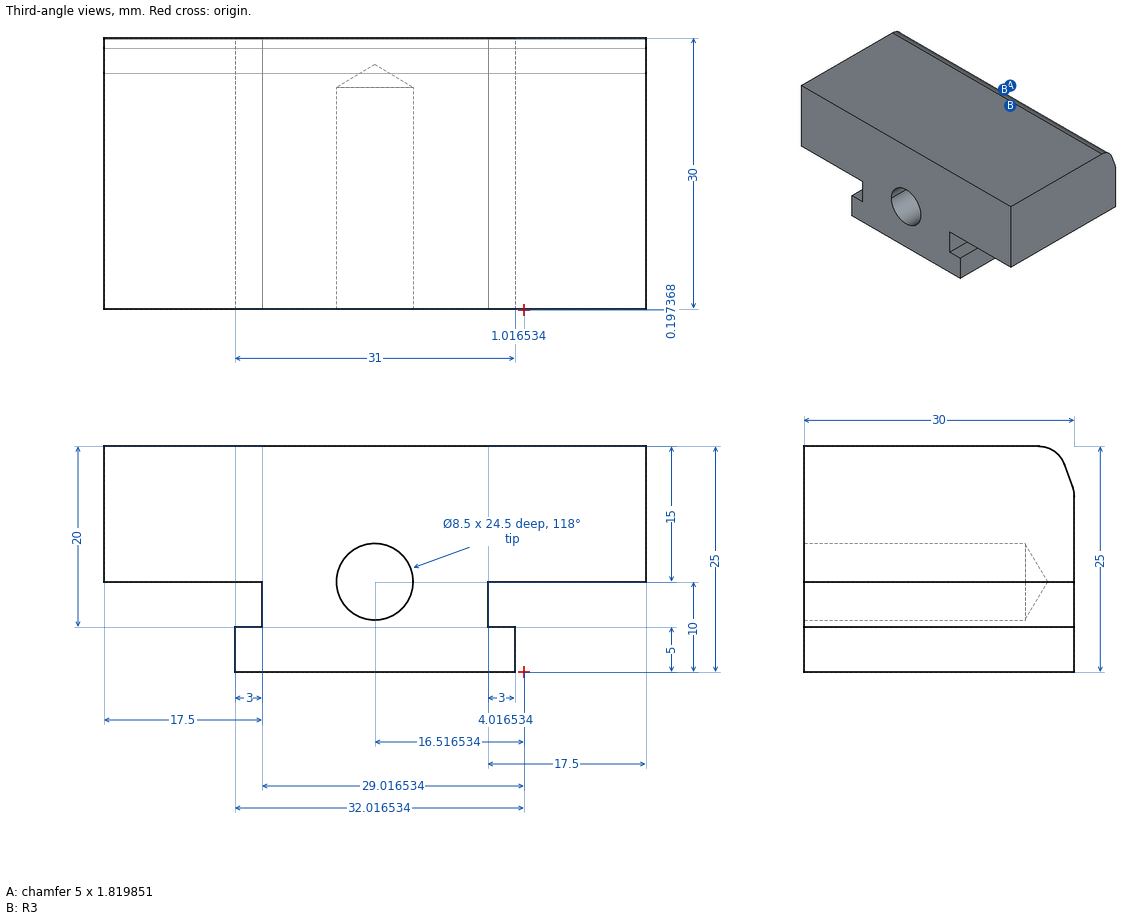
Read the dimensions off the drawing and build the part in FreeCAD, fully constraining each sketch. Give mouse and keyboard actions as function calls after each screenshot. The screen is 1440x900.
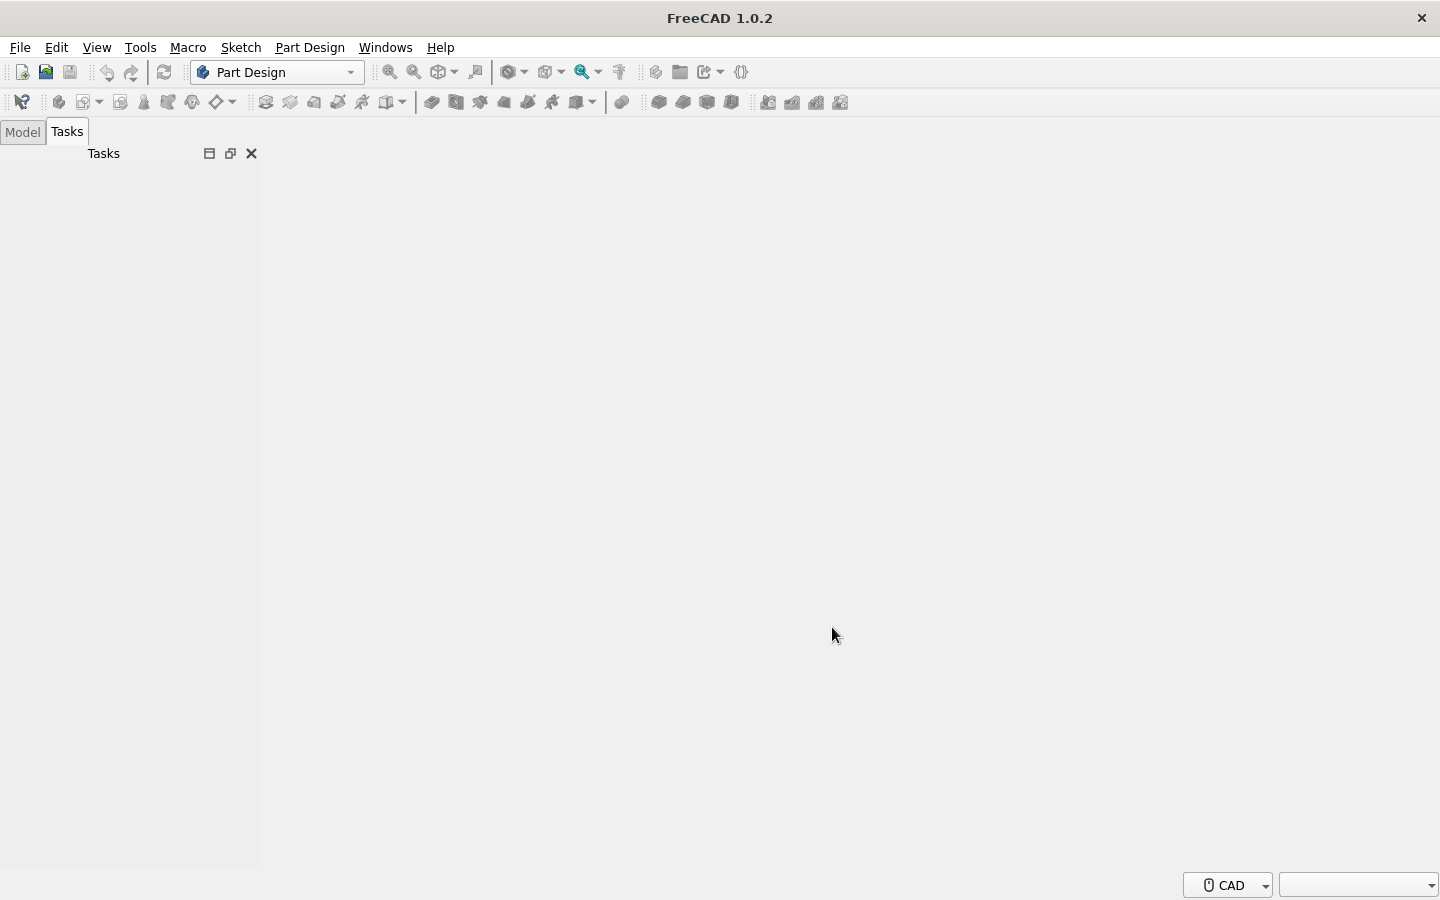
click(22, 72)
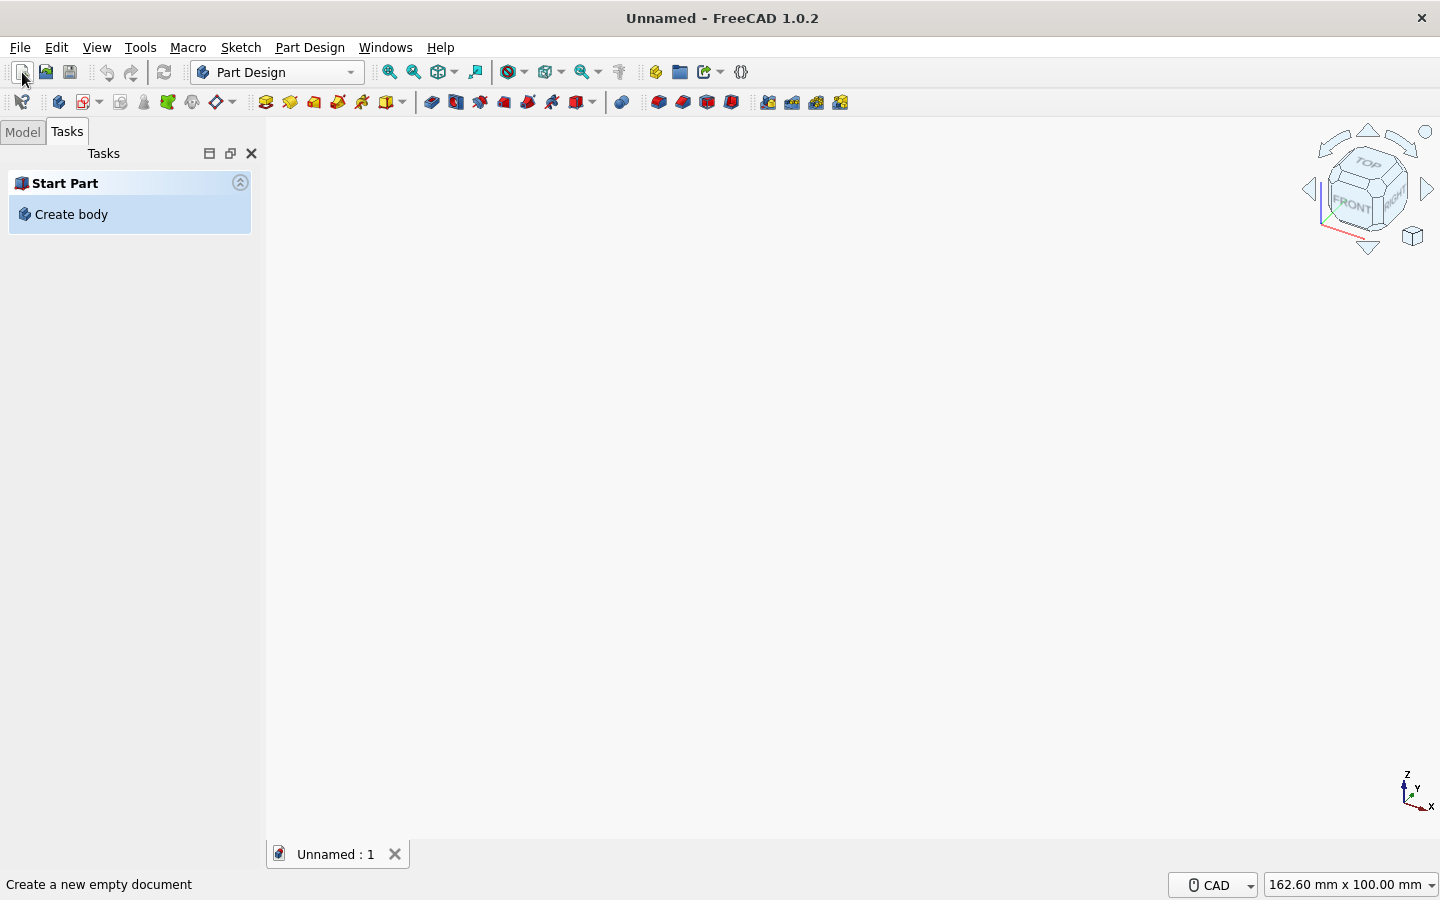
click(84, 102)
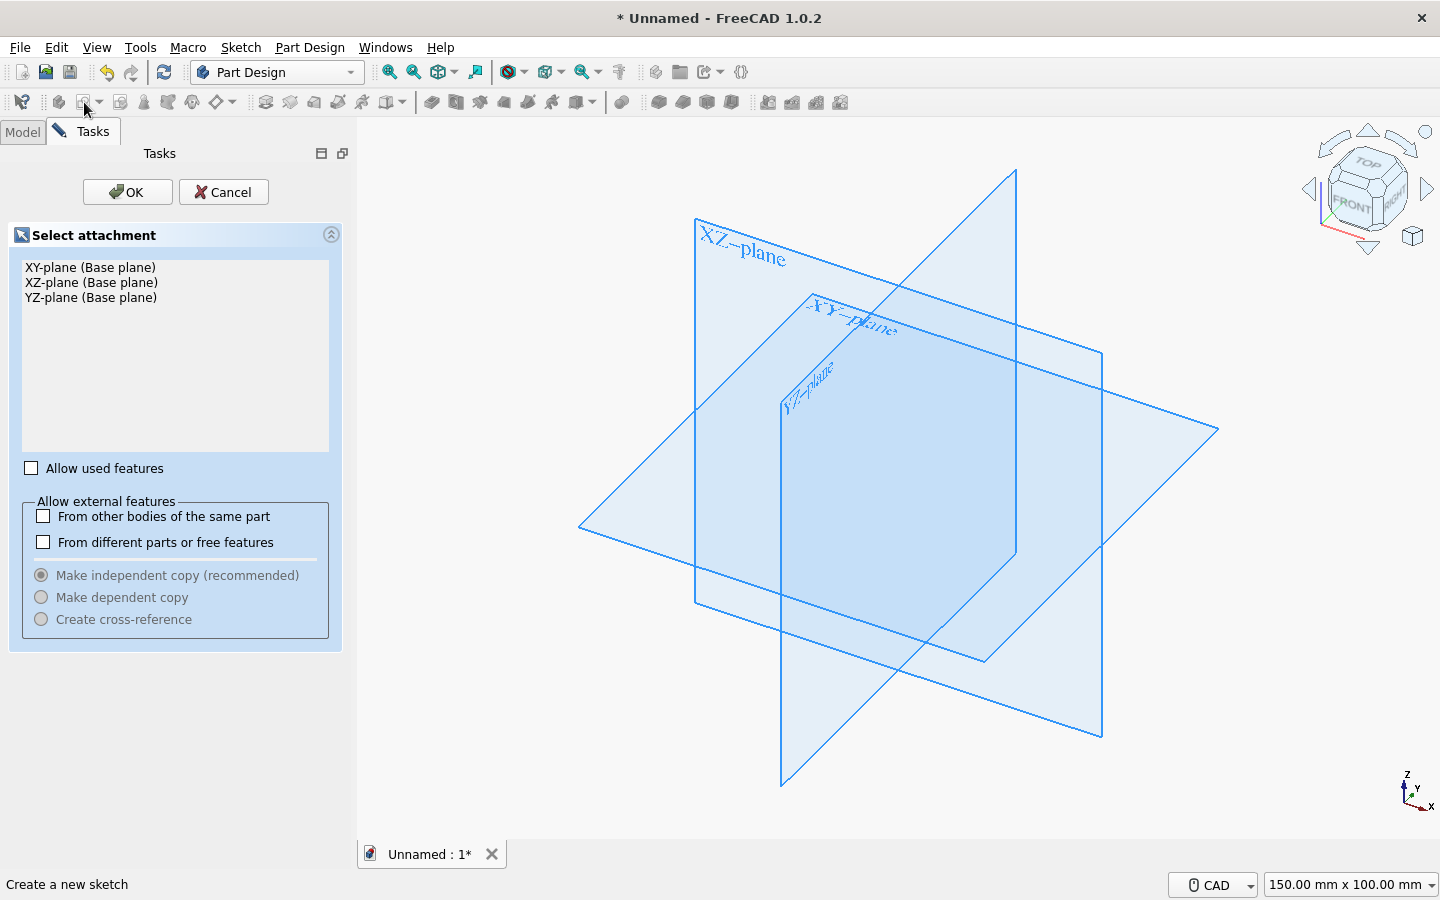
click(82, 268)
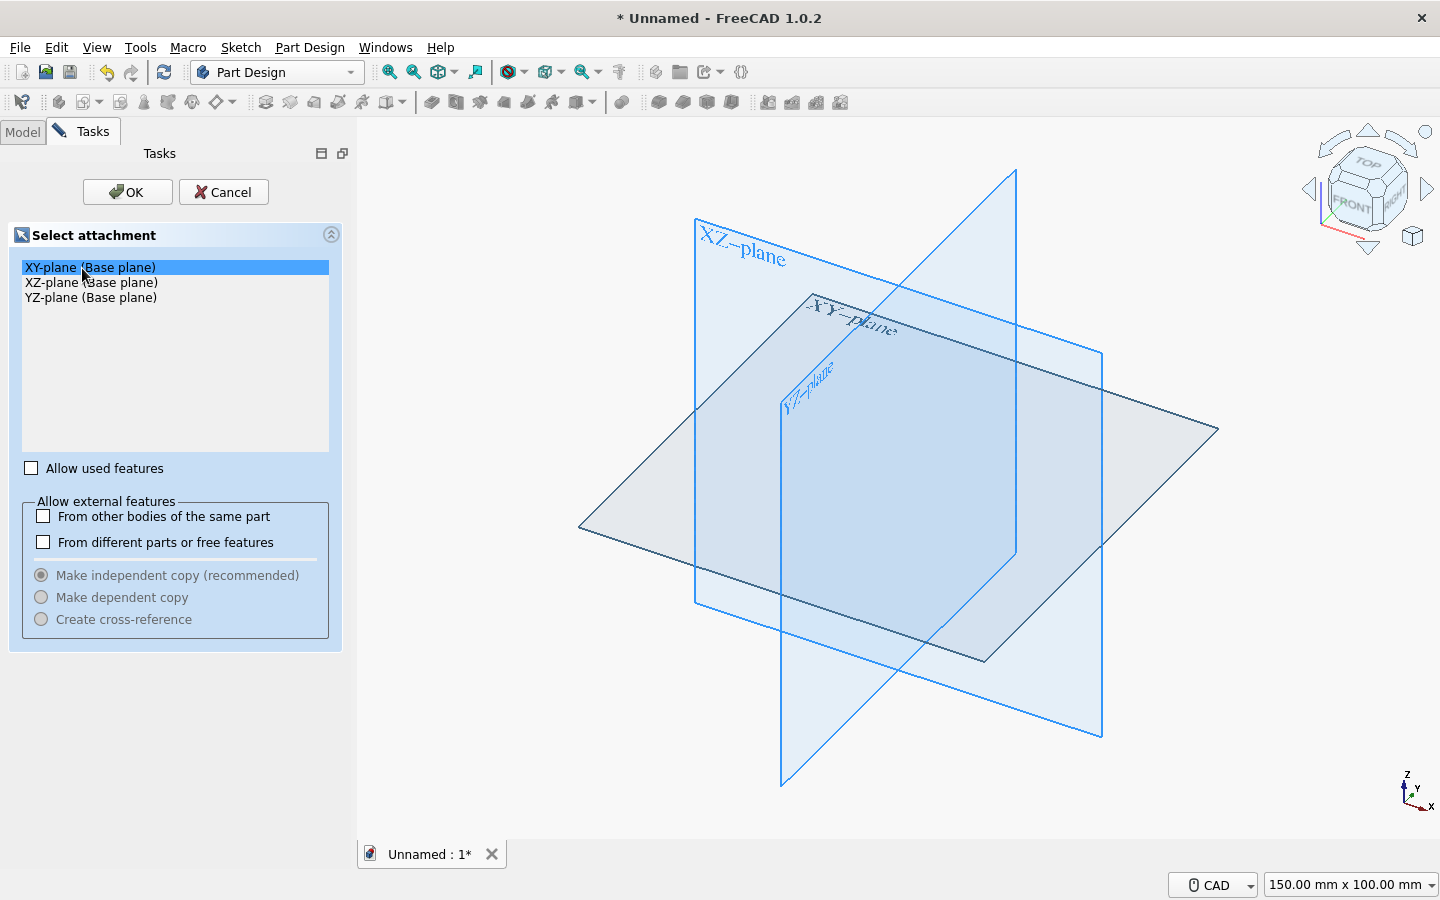
click(128, 192)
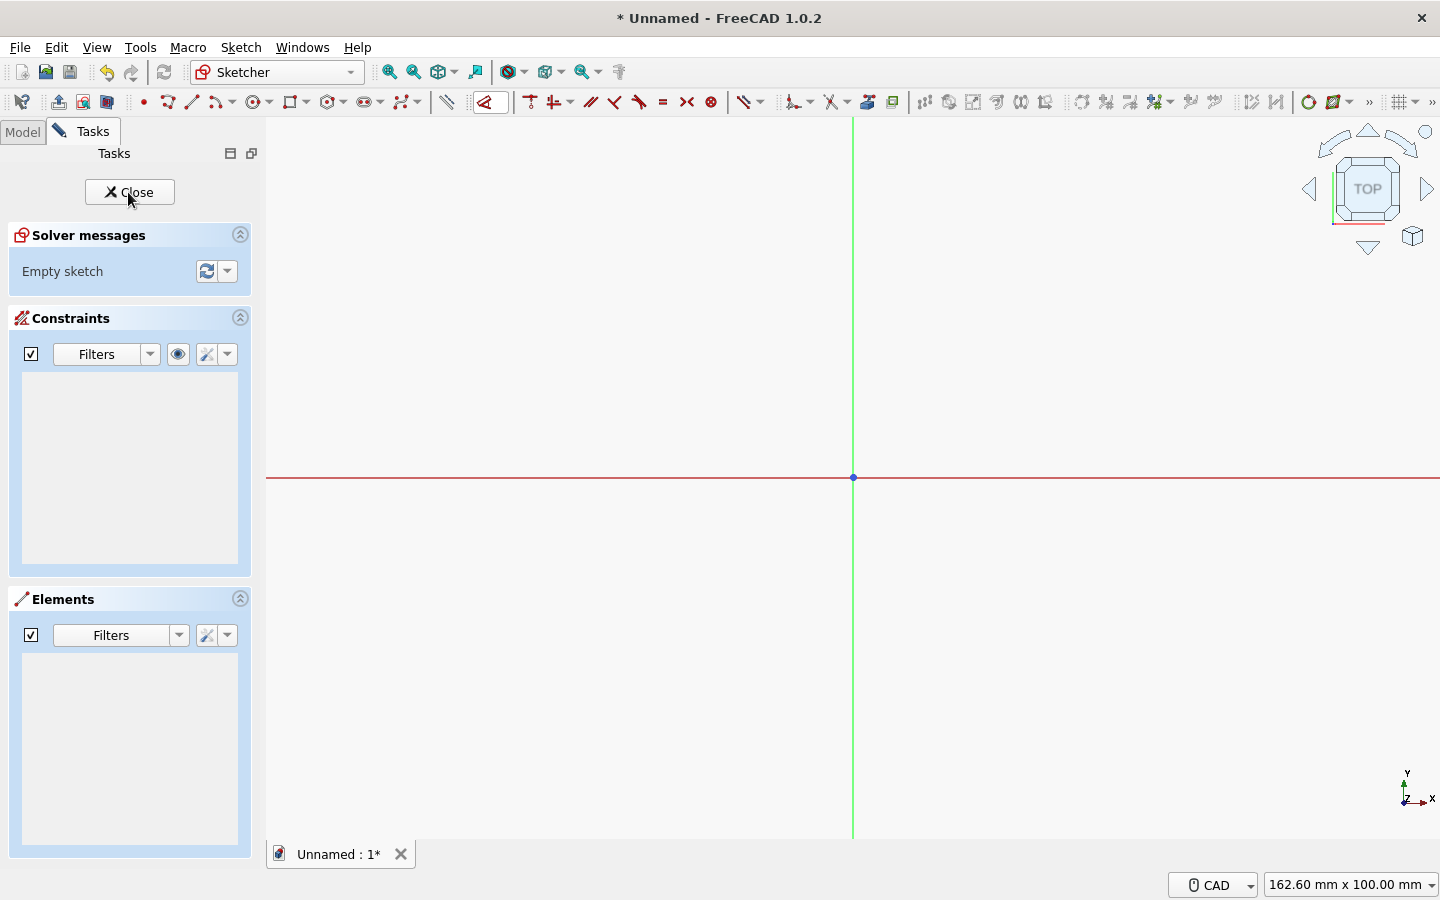
scroll(699, 280, up, 4)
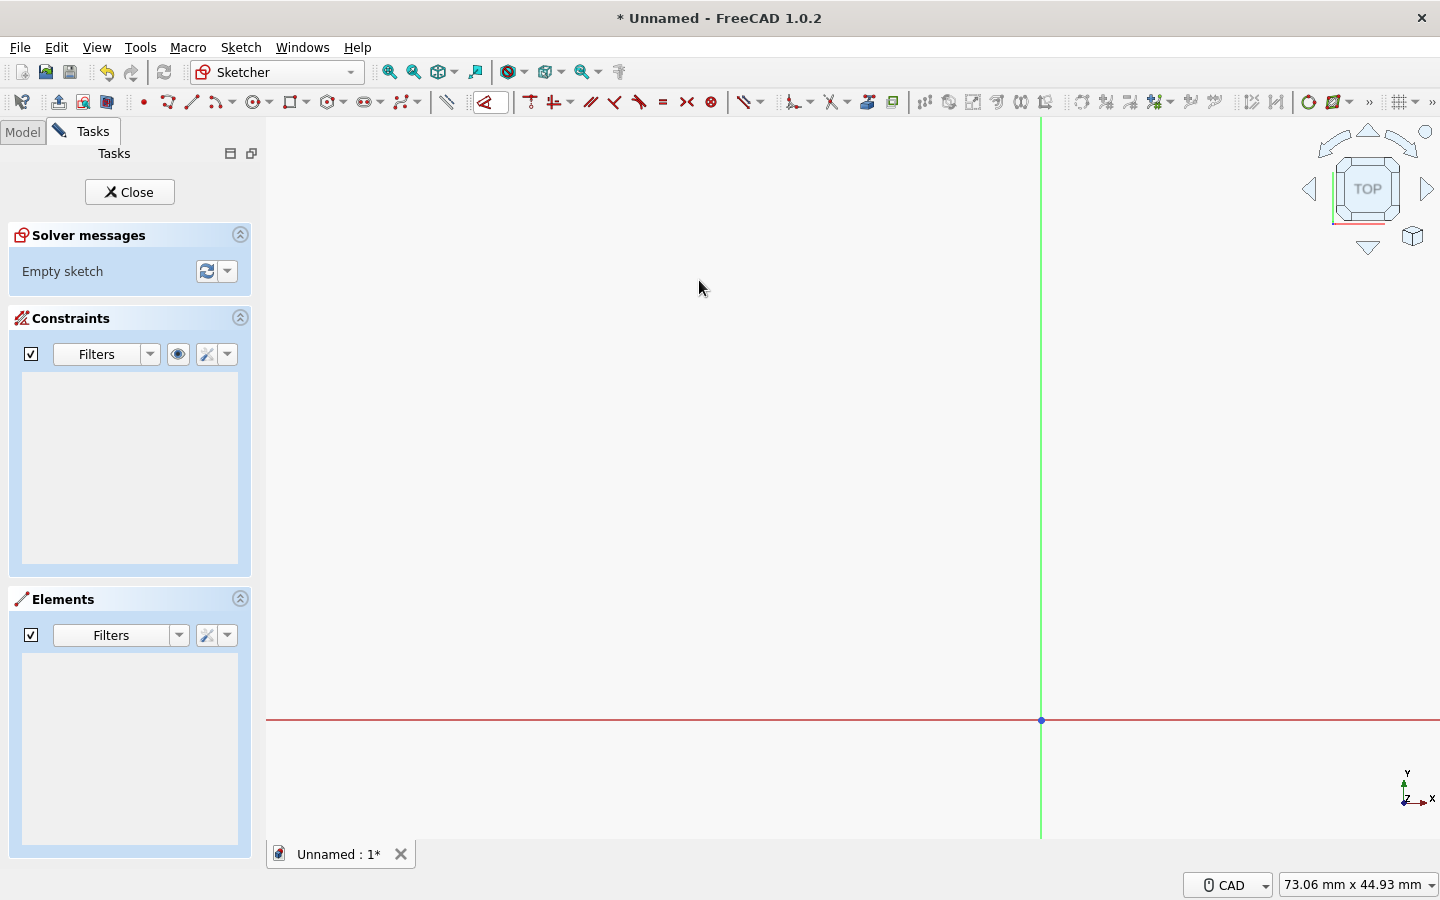
click(290, 102)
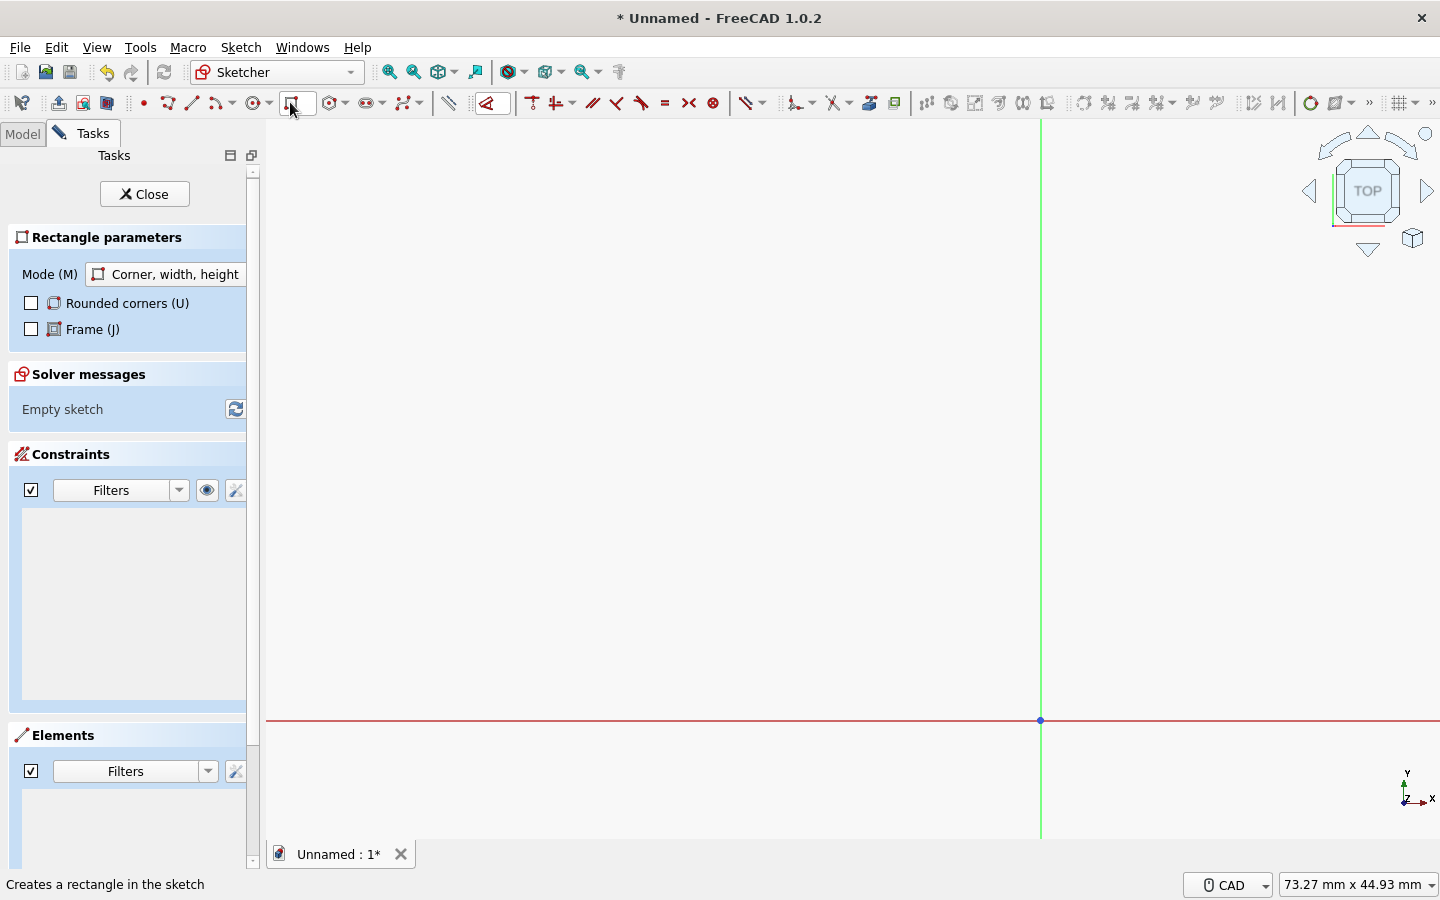
click(528, 237)